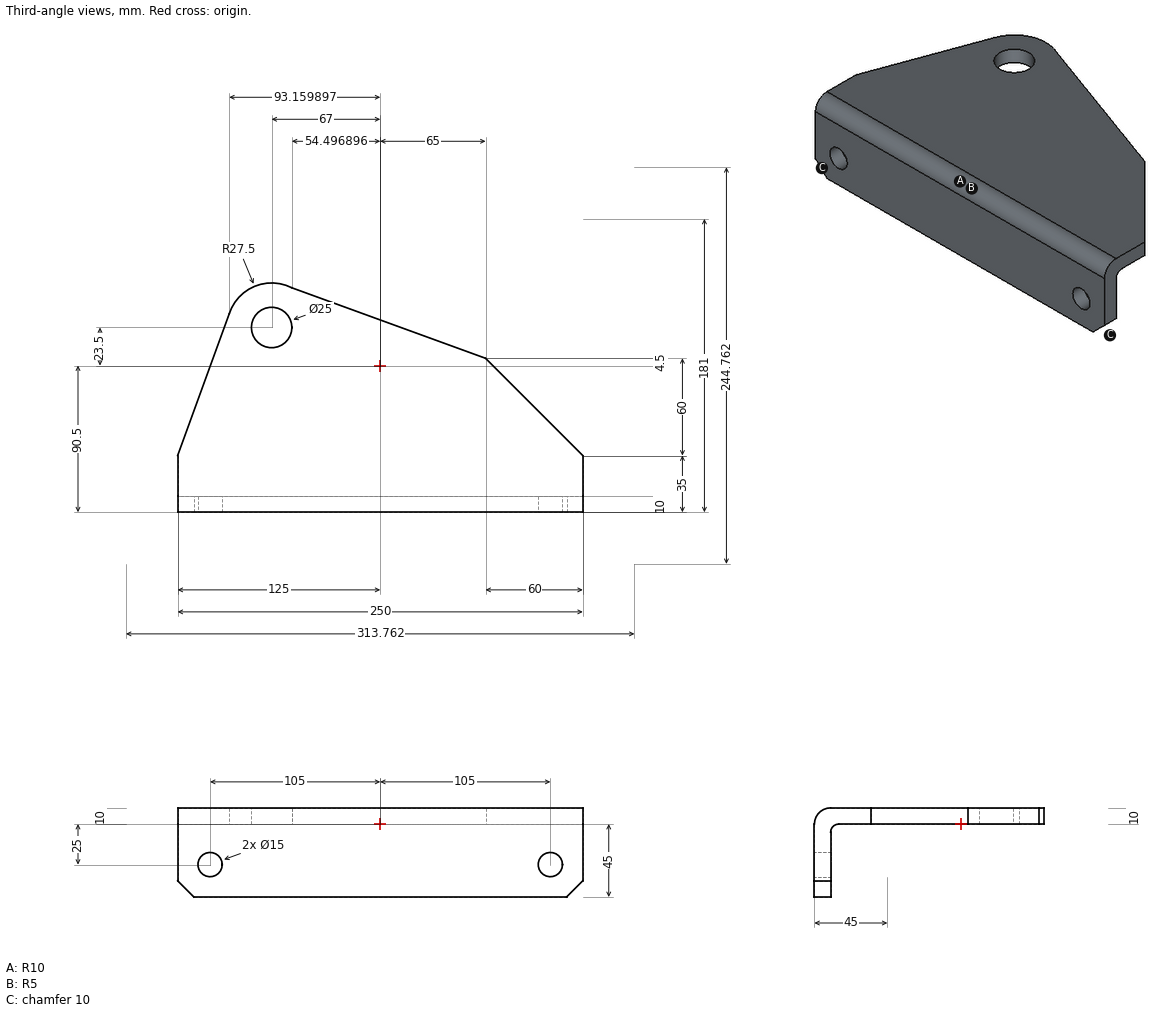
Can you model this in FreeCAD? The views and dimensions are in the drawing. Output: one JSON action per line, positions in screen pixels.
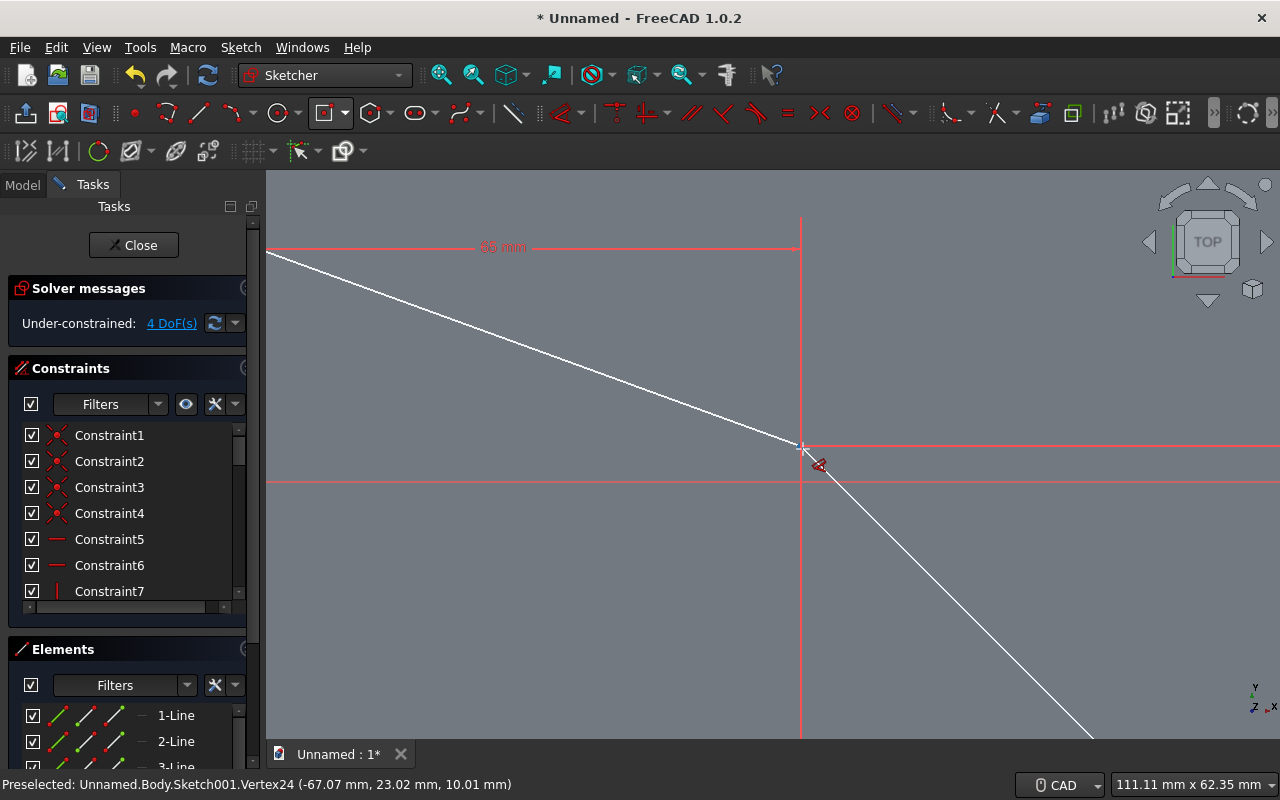
{"action": "left_click", "coordinate": [801, 446]}
{"action": "left_click", "coordinate": [835, 456]}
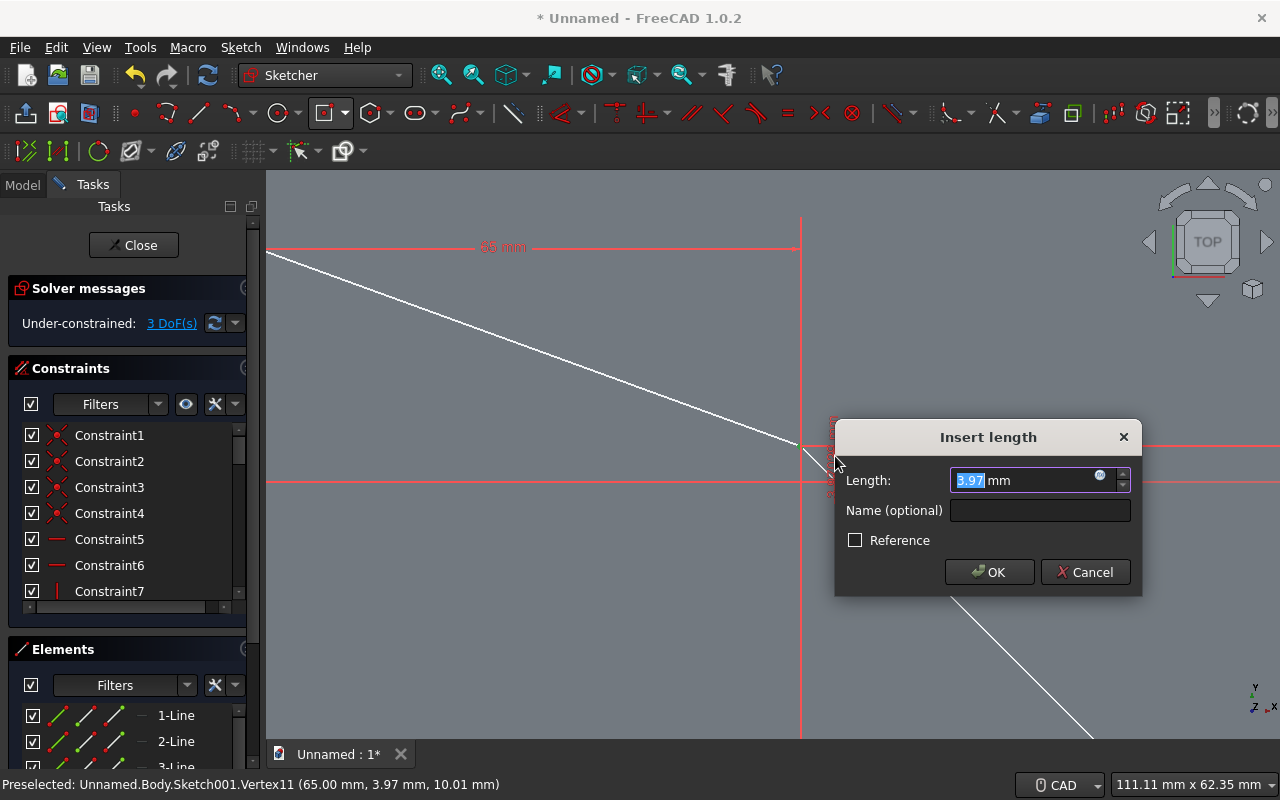
{"action": "type", "text": "4.5"}
{"action": "key", "text": "Return"}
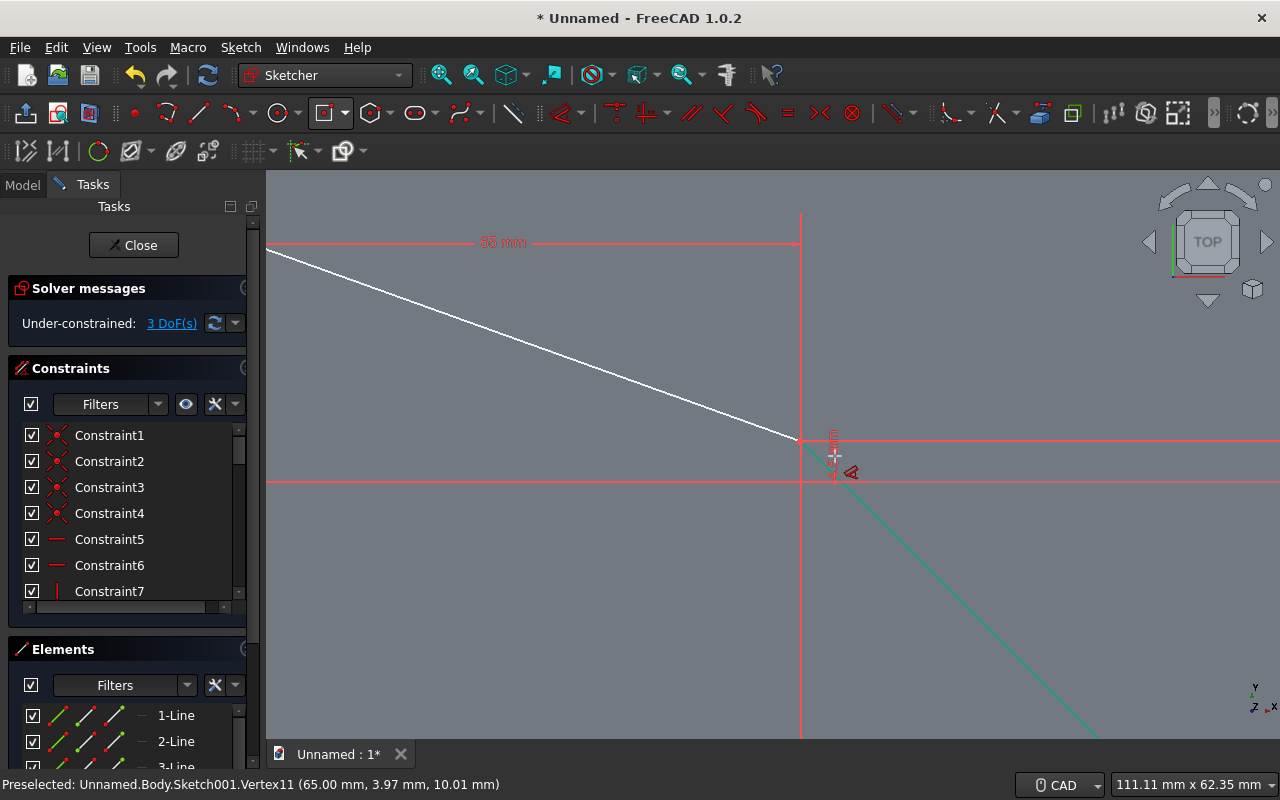
{"action": "scroll", "coordinate": [803, 449], "scroll_direction": "down", "scroll_amount": 9}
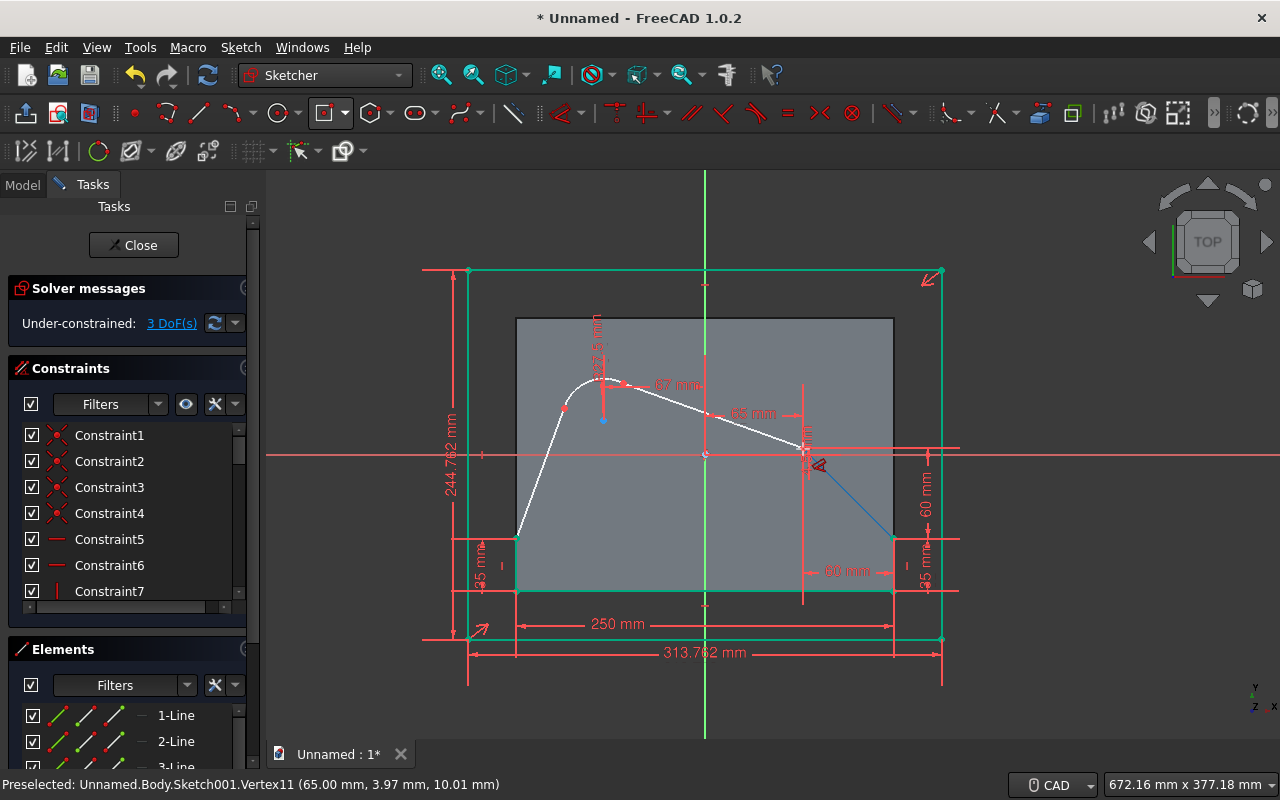
{"action": "left_click", "coordinate": [604, 420]}
{"action": "left_click", "coordinate": [570, 438]}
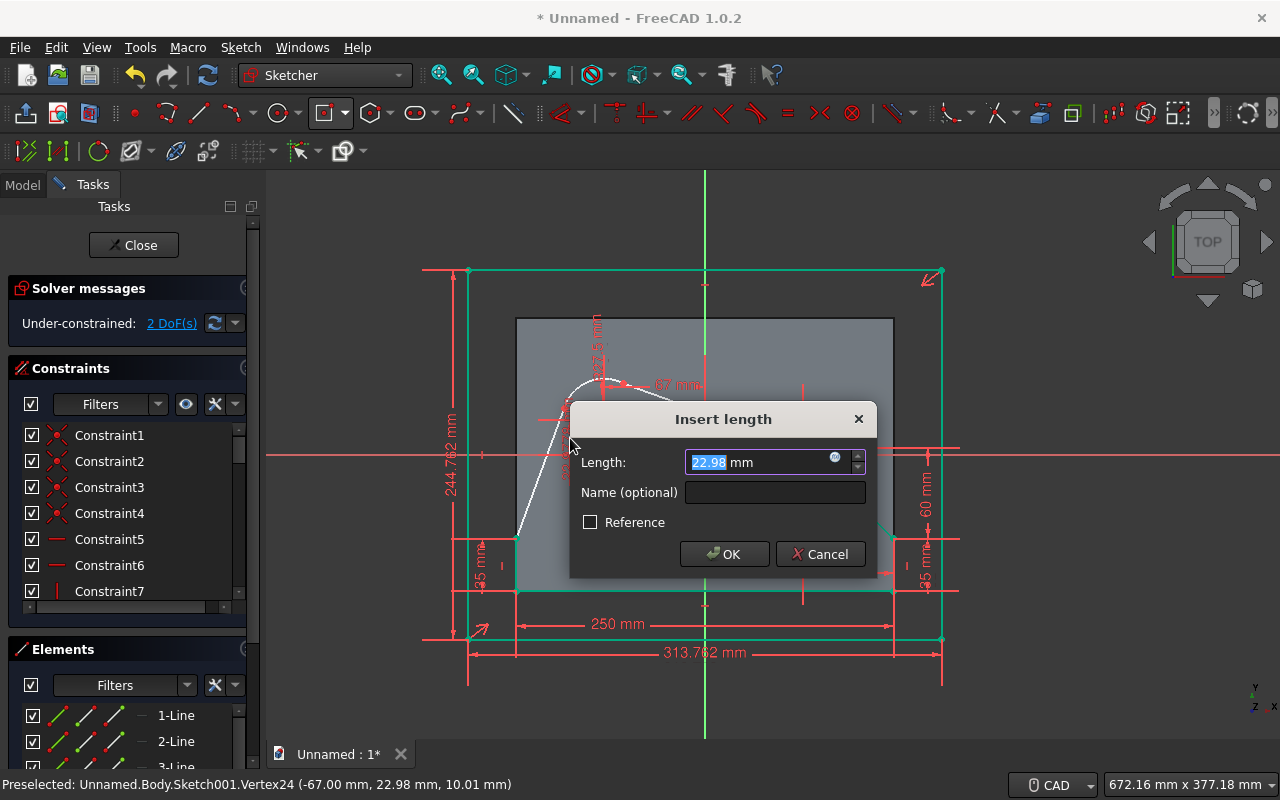
{"action": "type", "text": "23.5"}
{"action": "key", "text": "Return"}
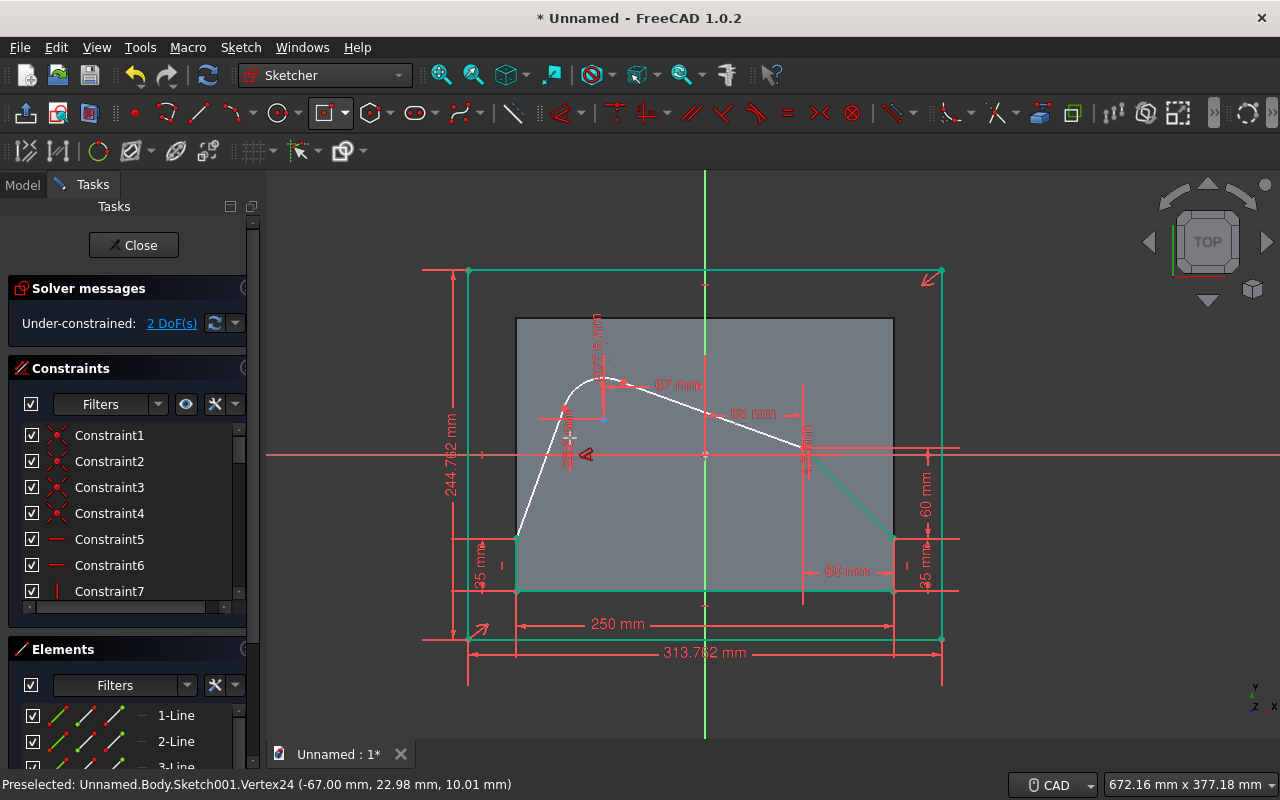
{"action": "left_click", "coordinate": [623, 383]}
{"action": "left_click", "coordinate": [683, 349]}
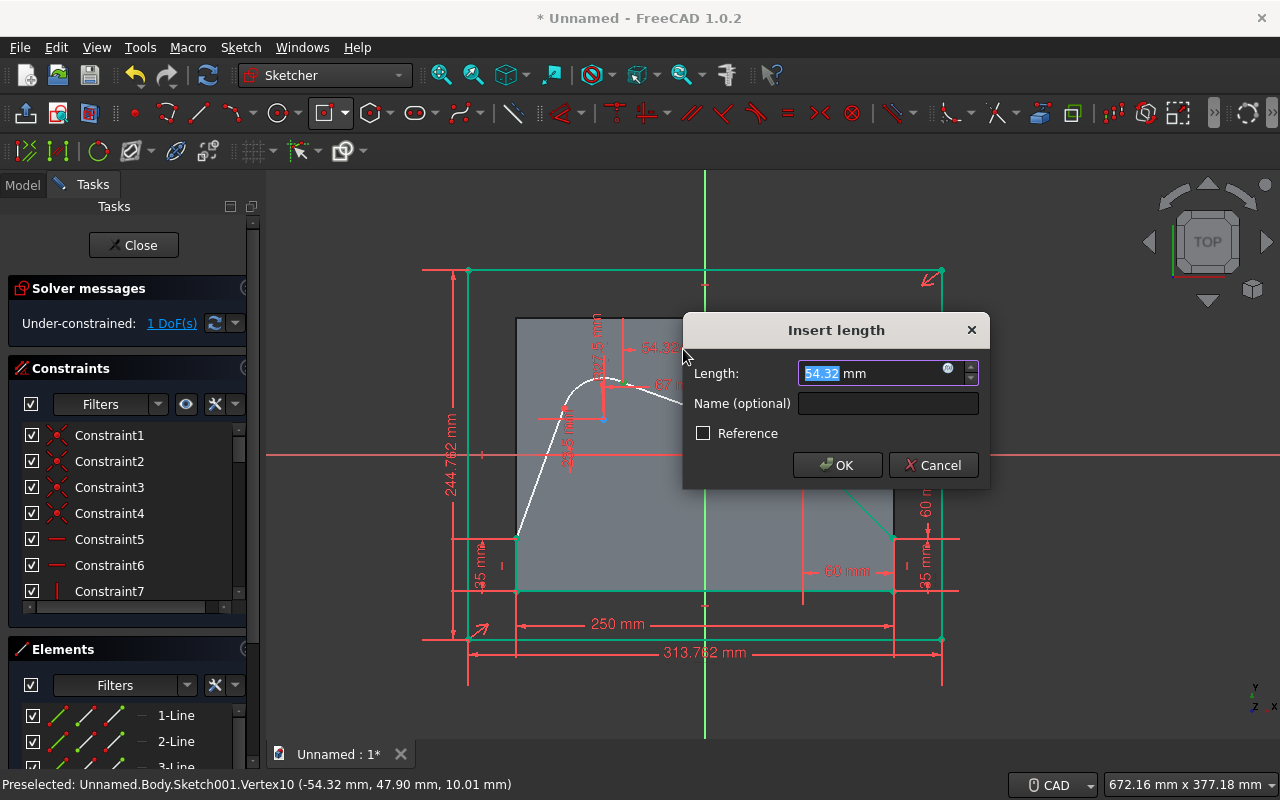
{"action": "type", "text": "54.496896"}
{"action": "key", "text": "Return"}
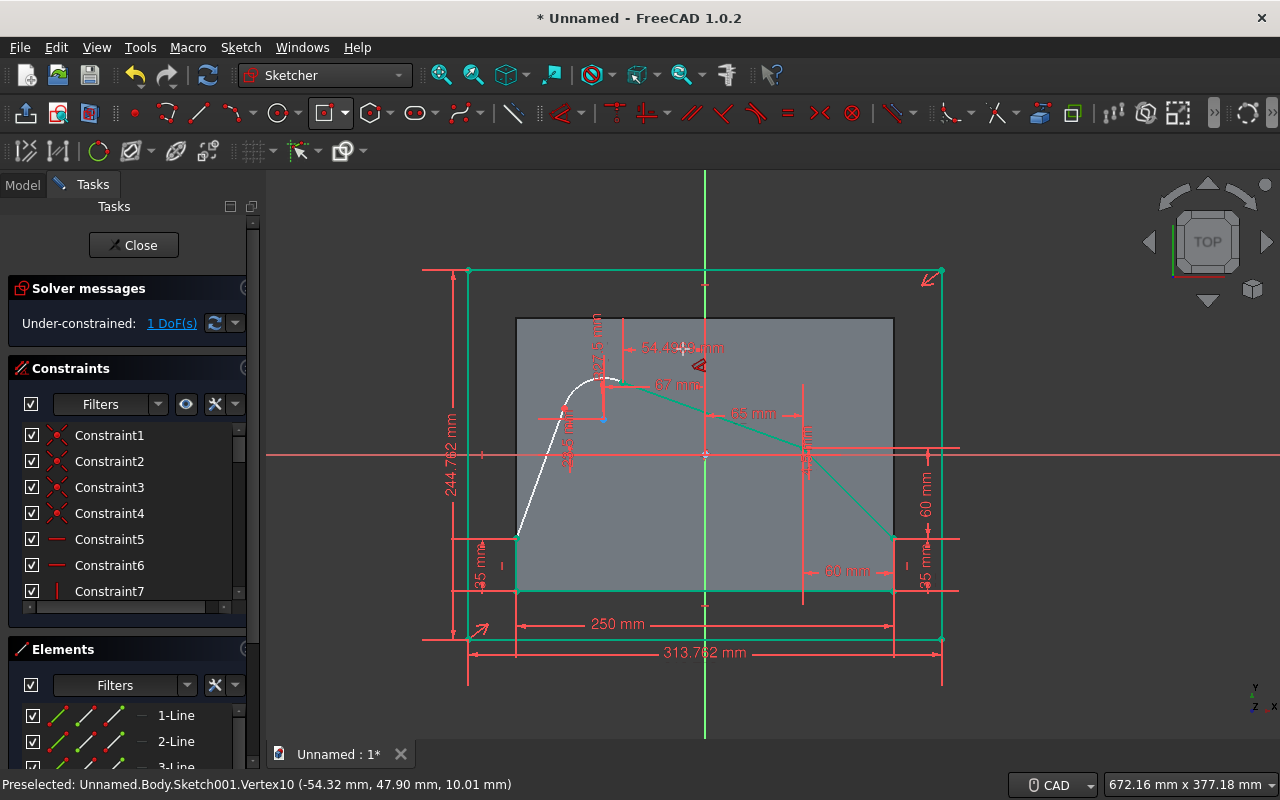
{"action": "left_click", "coordinate": [564, 408]}
{"action": "left_click", "coordinate": [635, 489]}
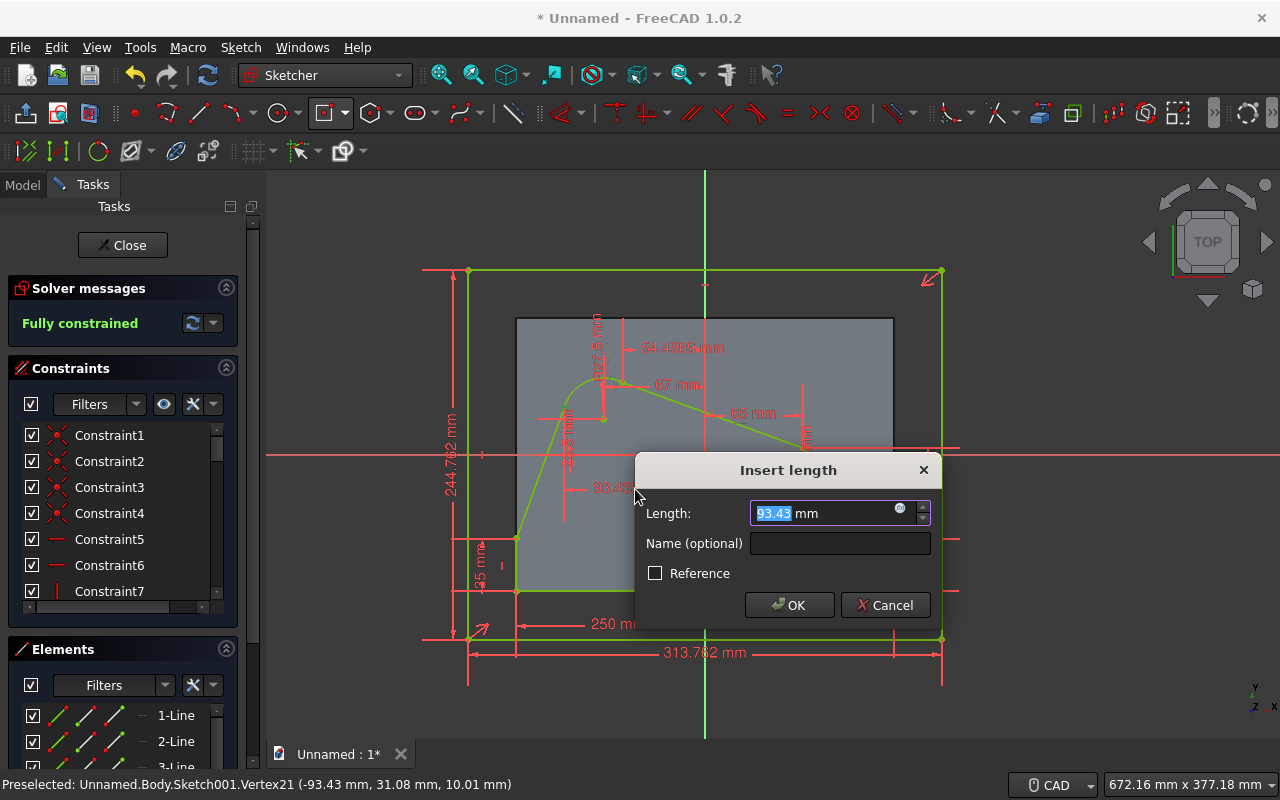
{"action": "type", "text": "93.159897"}
{"action": "key", "text": "Return"}
{"action": "key", "text": "Escape"}